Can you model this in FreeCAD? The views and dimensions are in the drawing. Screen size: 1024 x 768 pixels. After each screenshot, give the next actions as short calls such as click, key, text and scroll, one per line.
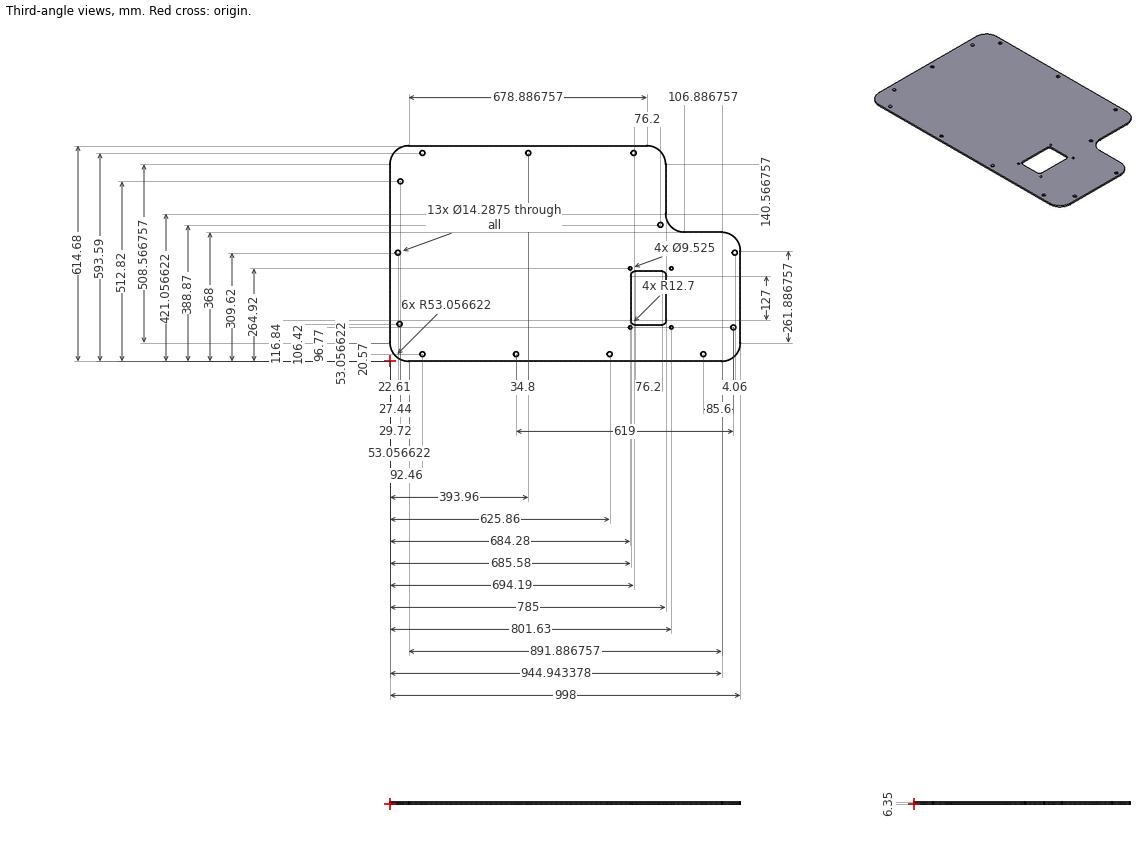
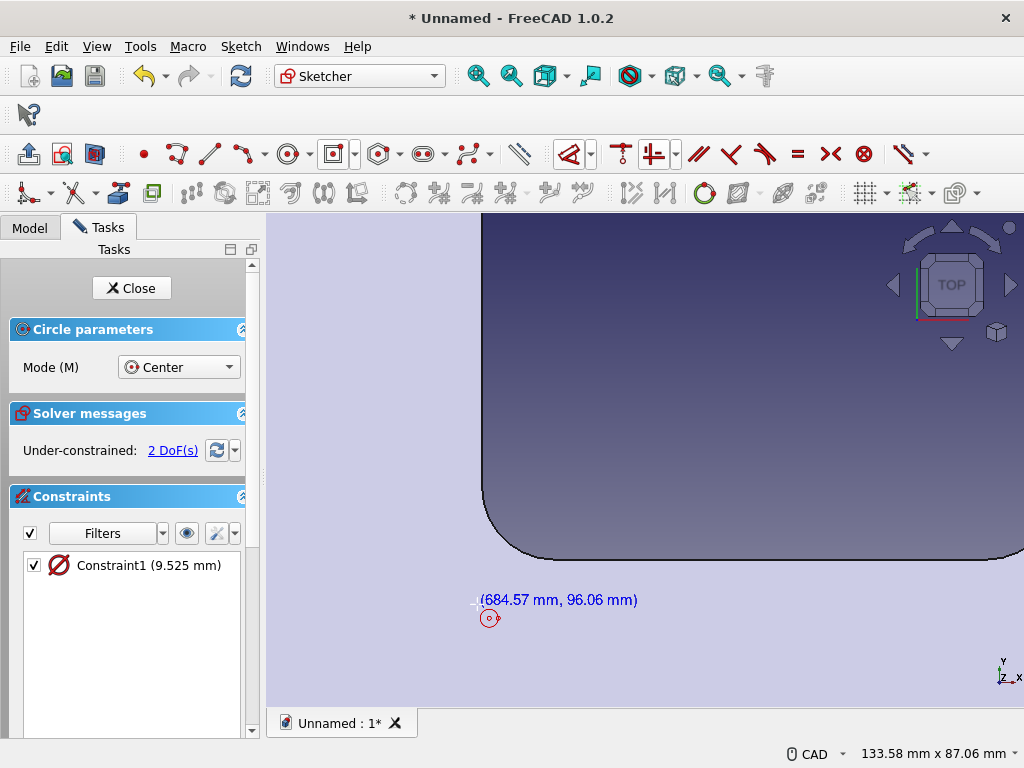
click(475, 601)
move(494, 582)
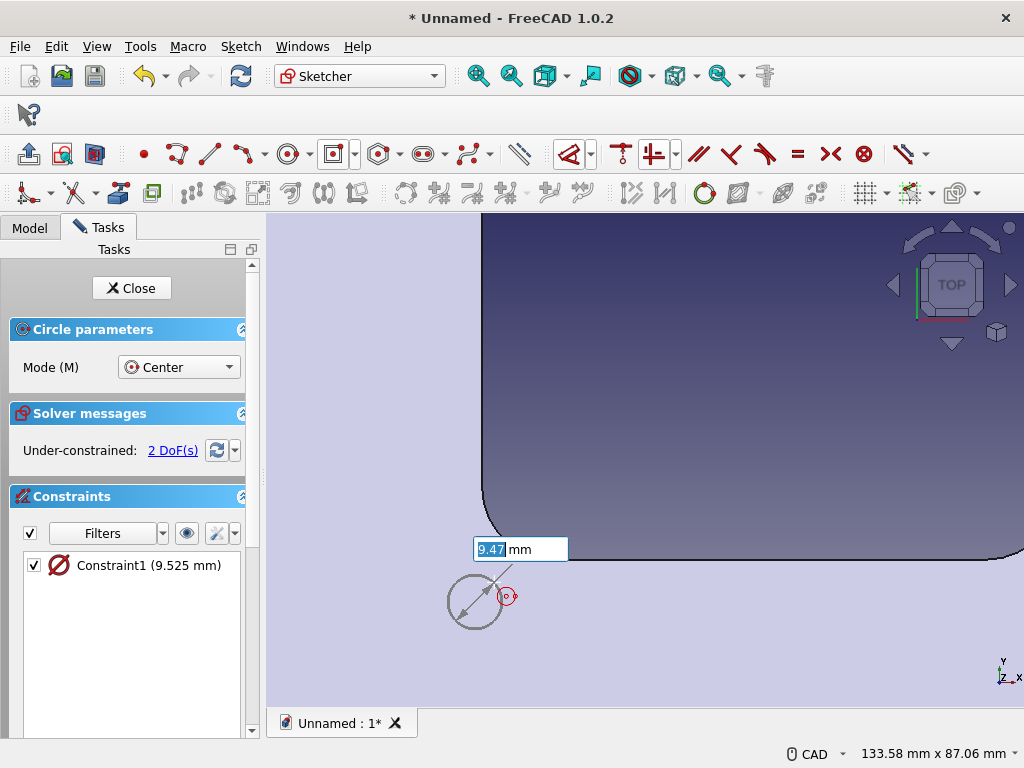
text(9.525)
key(Return)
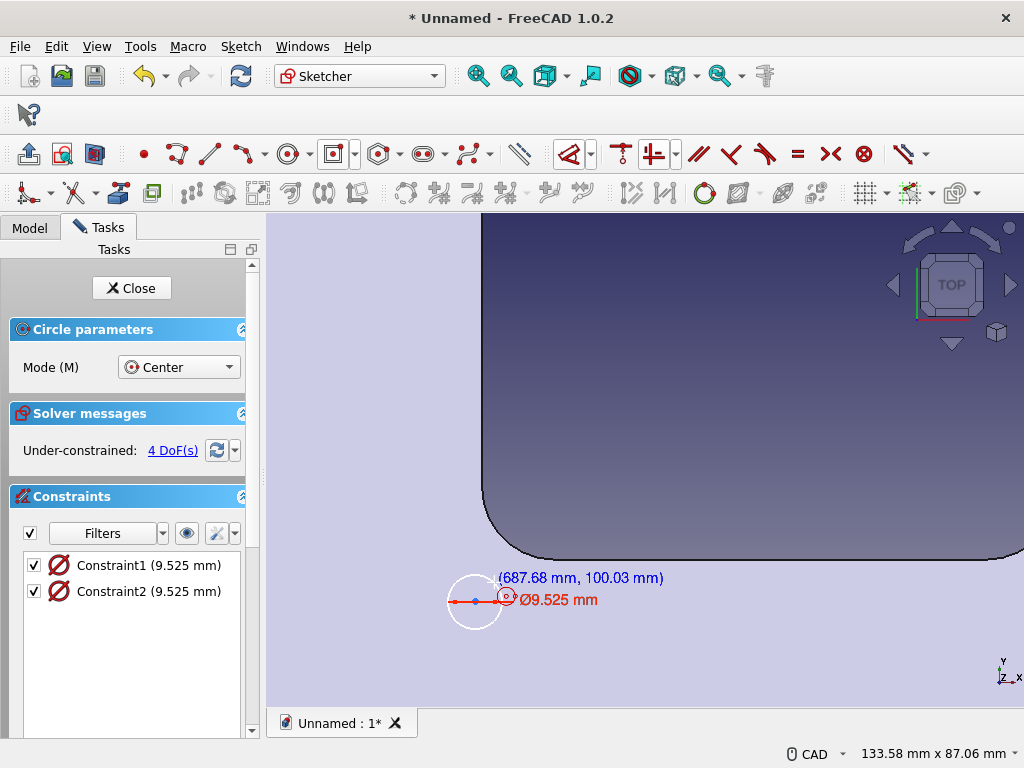
scroll(477, 605, down, 6)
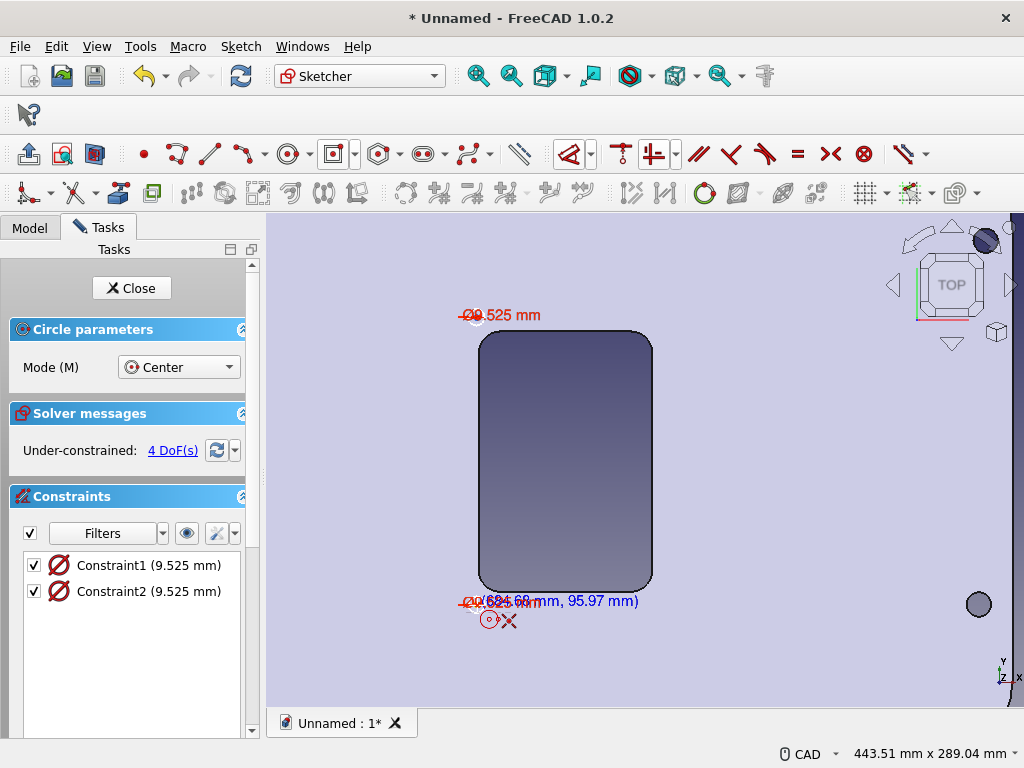
scroll(677, 604, up, 6)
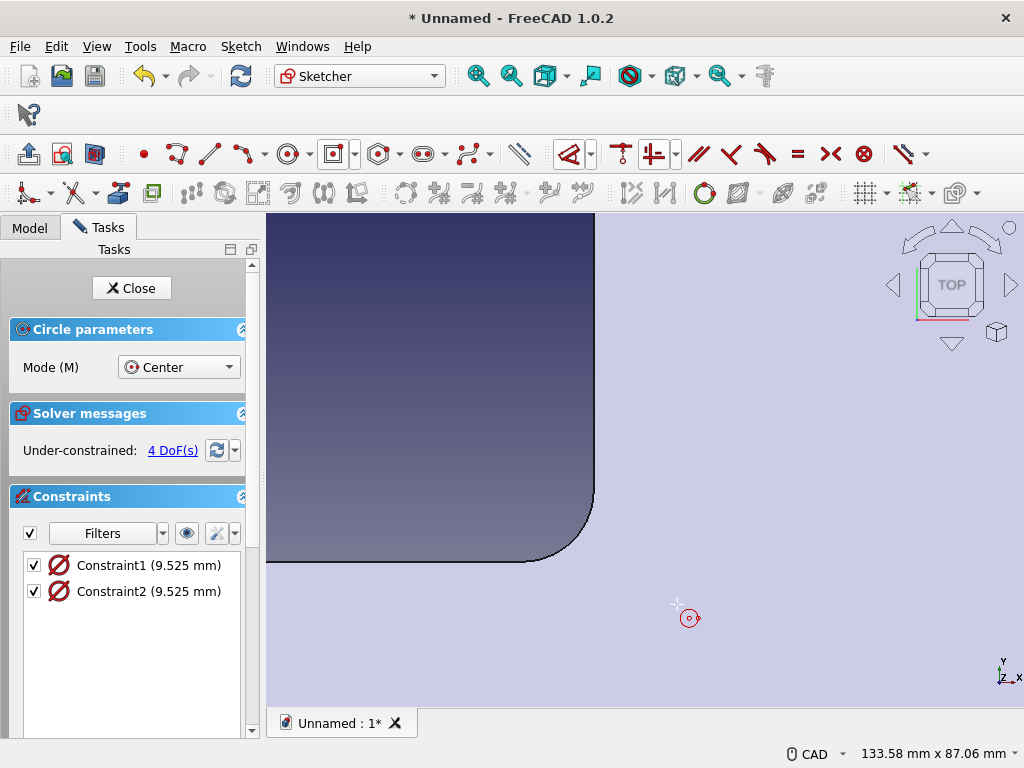
click(676, 604)
move(695, 585)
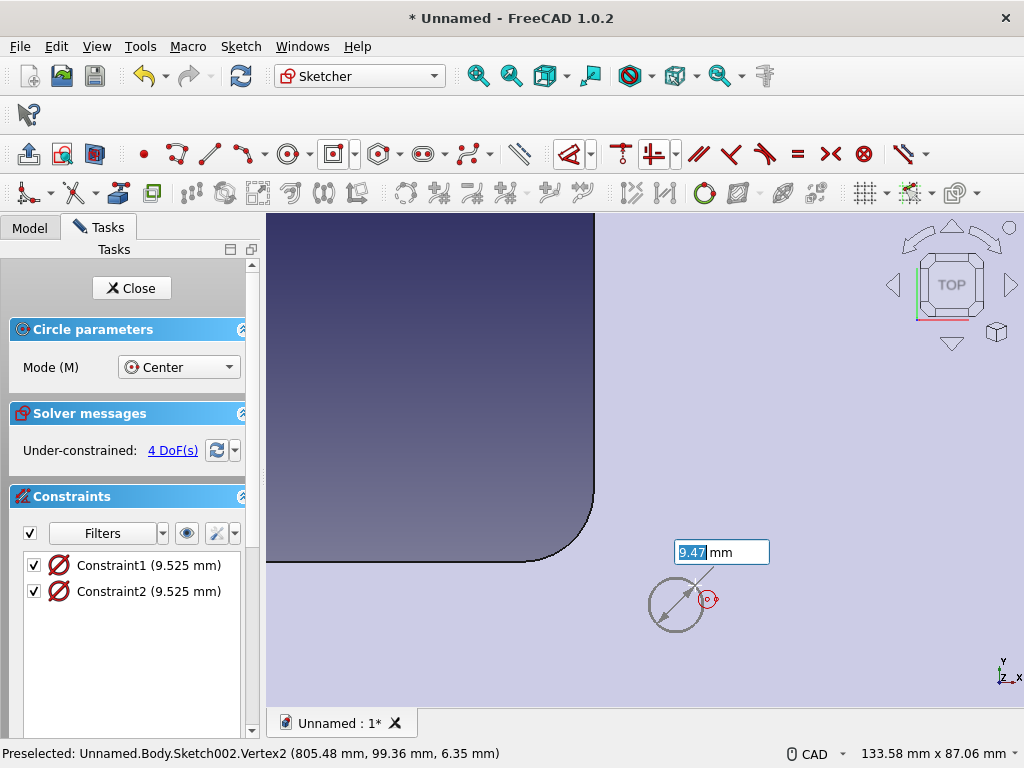
text(9.525)
key(Return)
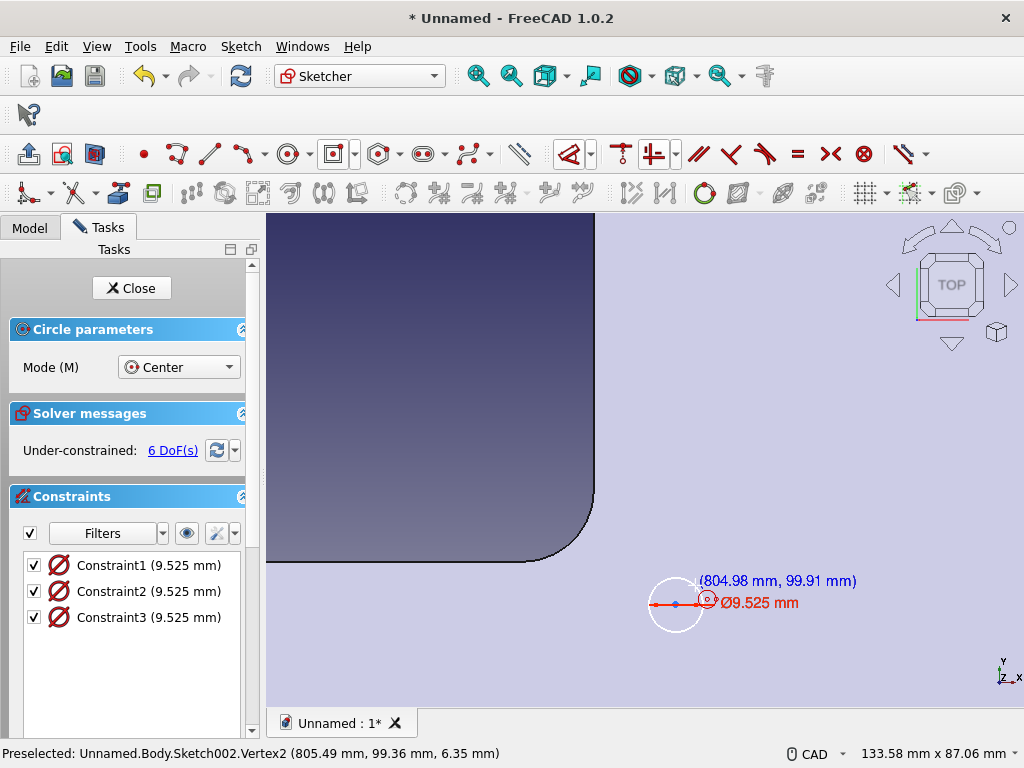
scroll(677, 604, down, 6)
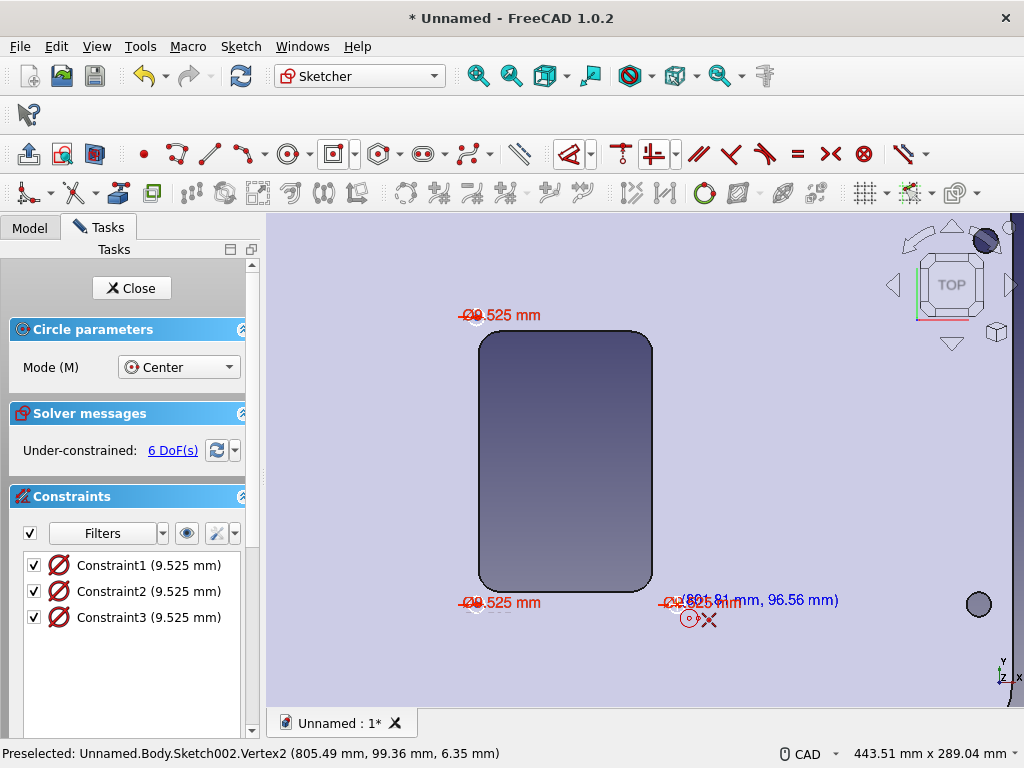
scroll(677, 317, up, 6)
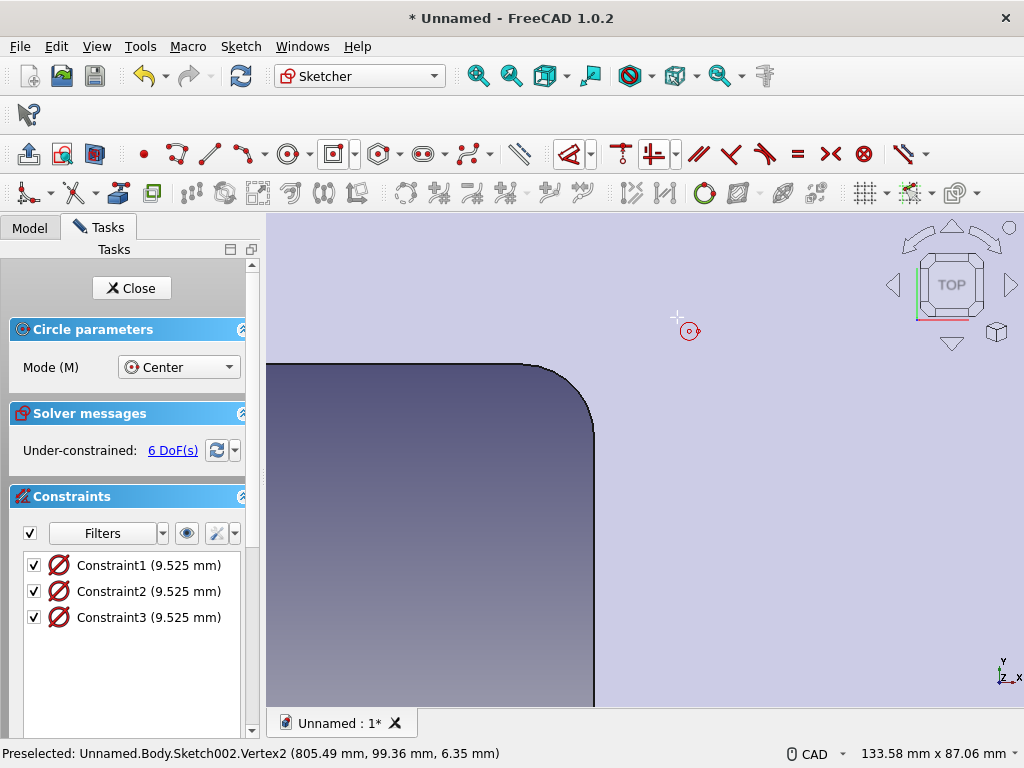
click(676, 317)
move(695, 298)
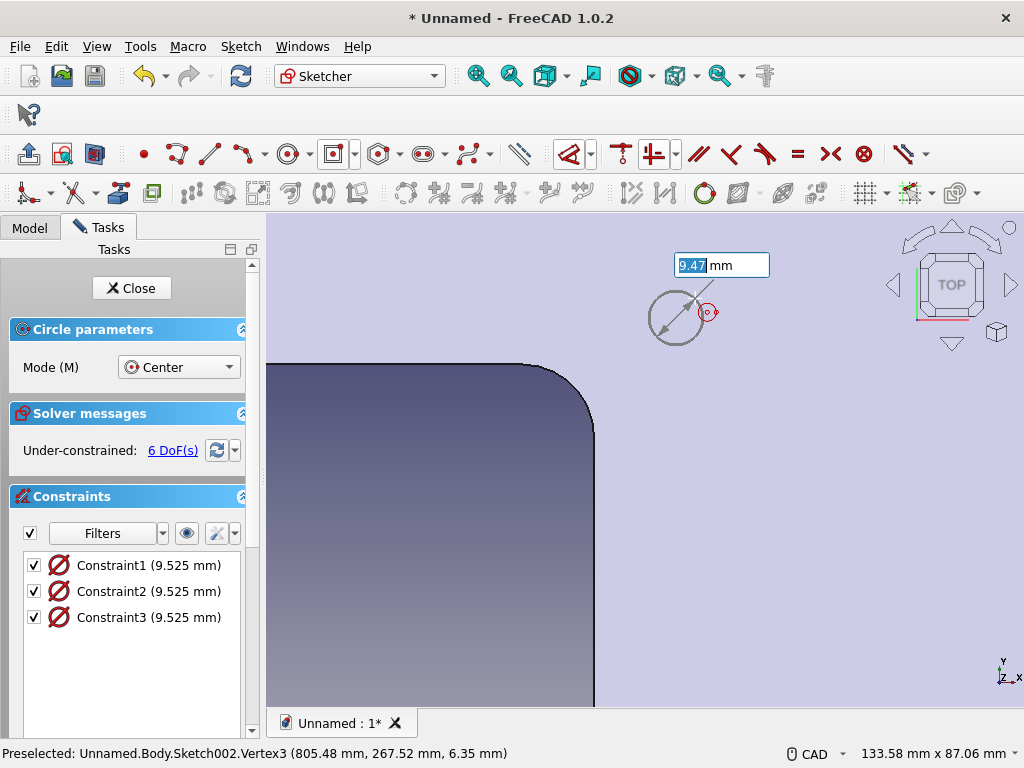
text(9.525)
key(Return)
key(Escape)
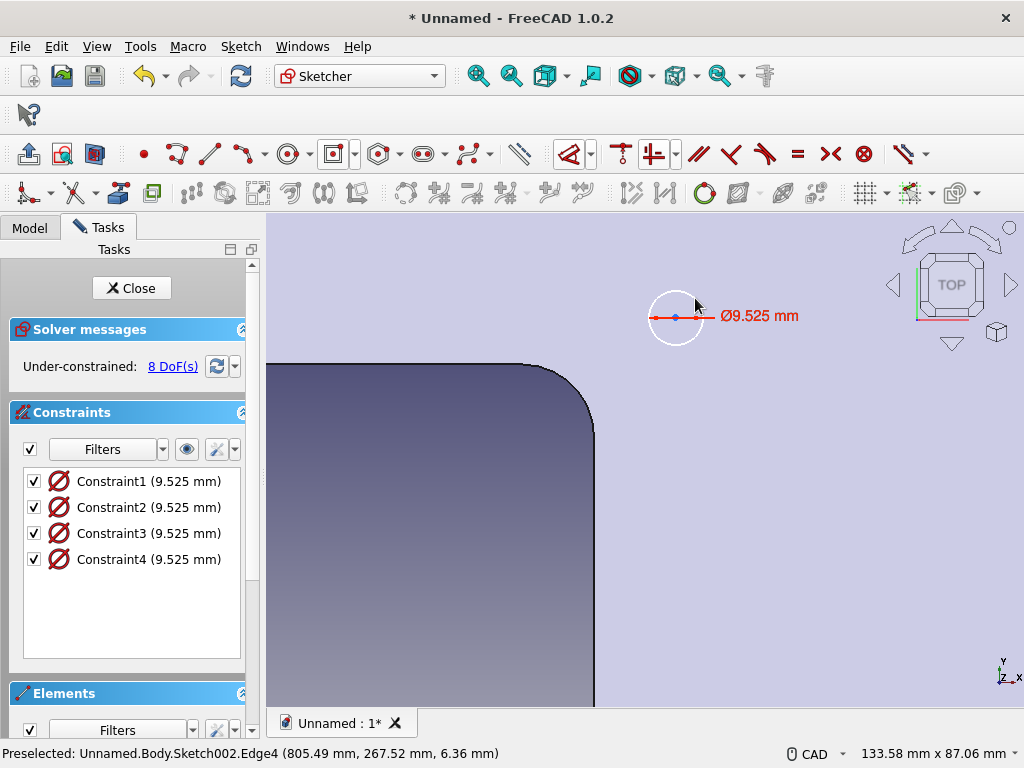
scroll(677, 316, down, 6)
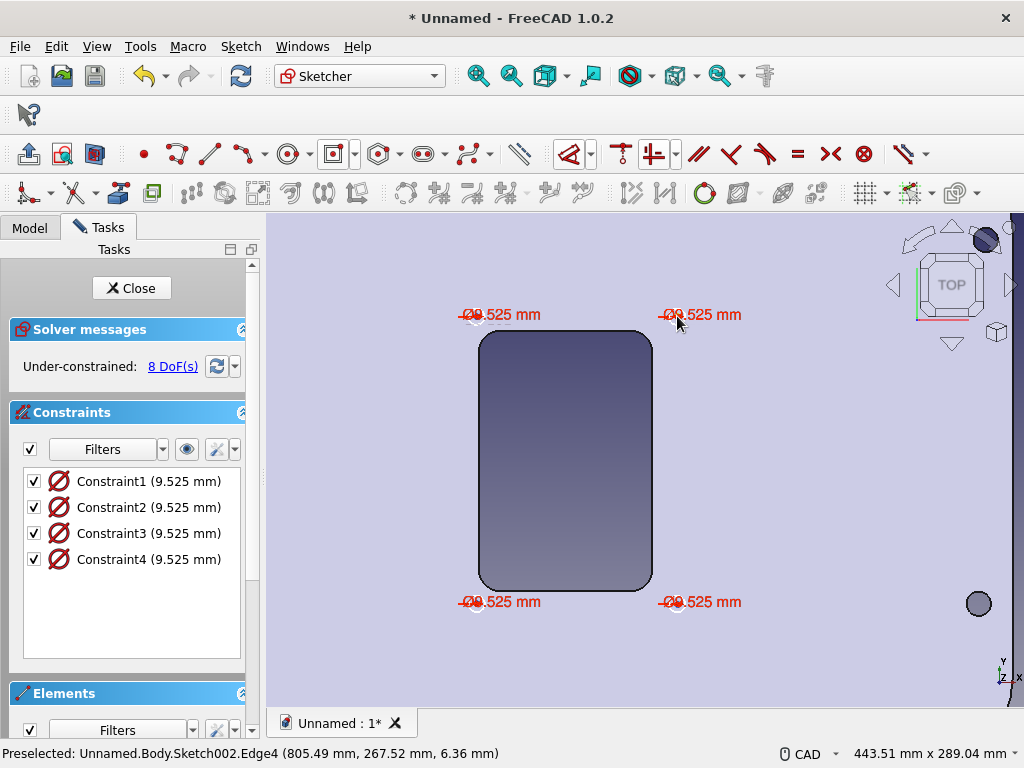
click(477, 604)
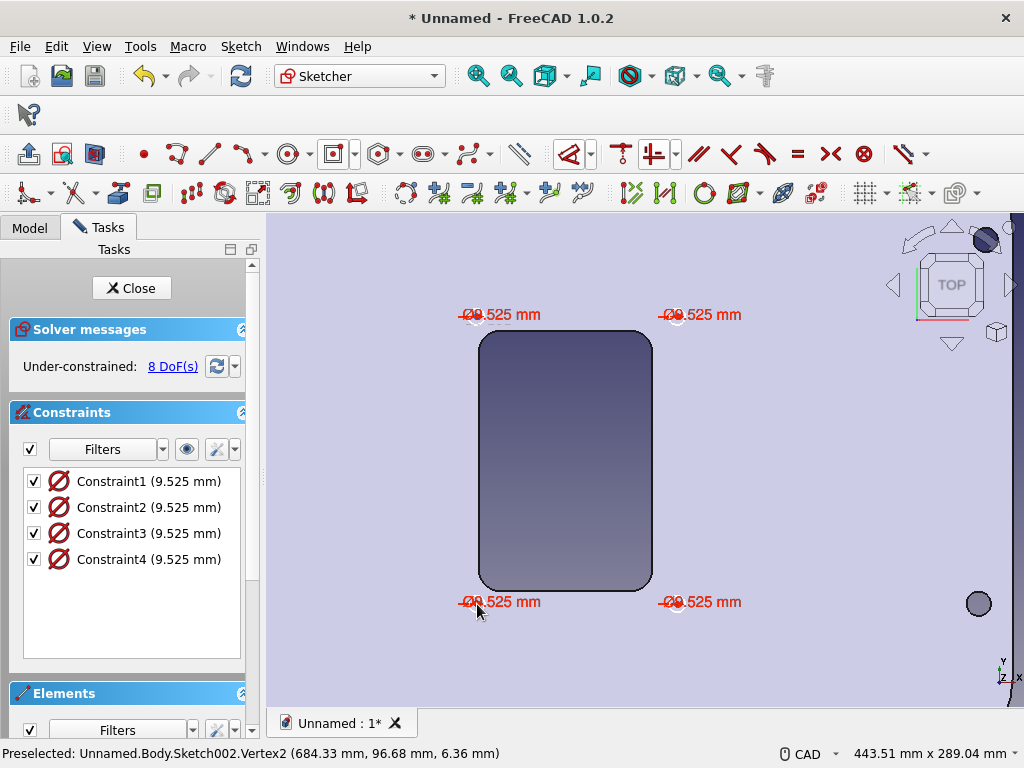
click(590, 154)